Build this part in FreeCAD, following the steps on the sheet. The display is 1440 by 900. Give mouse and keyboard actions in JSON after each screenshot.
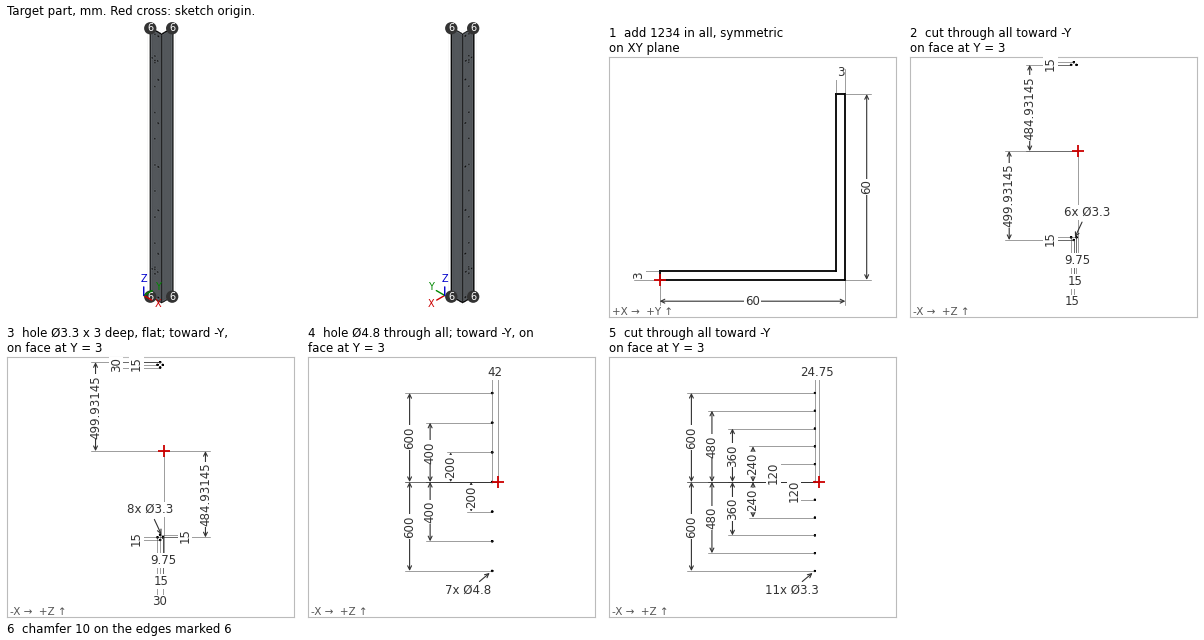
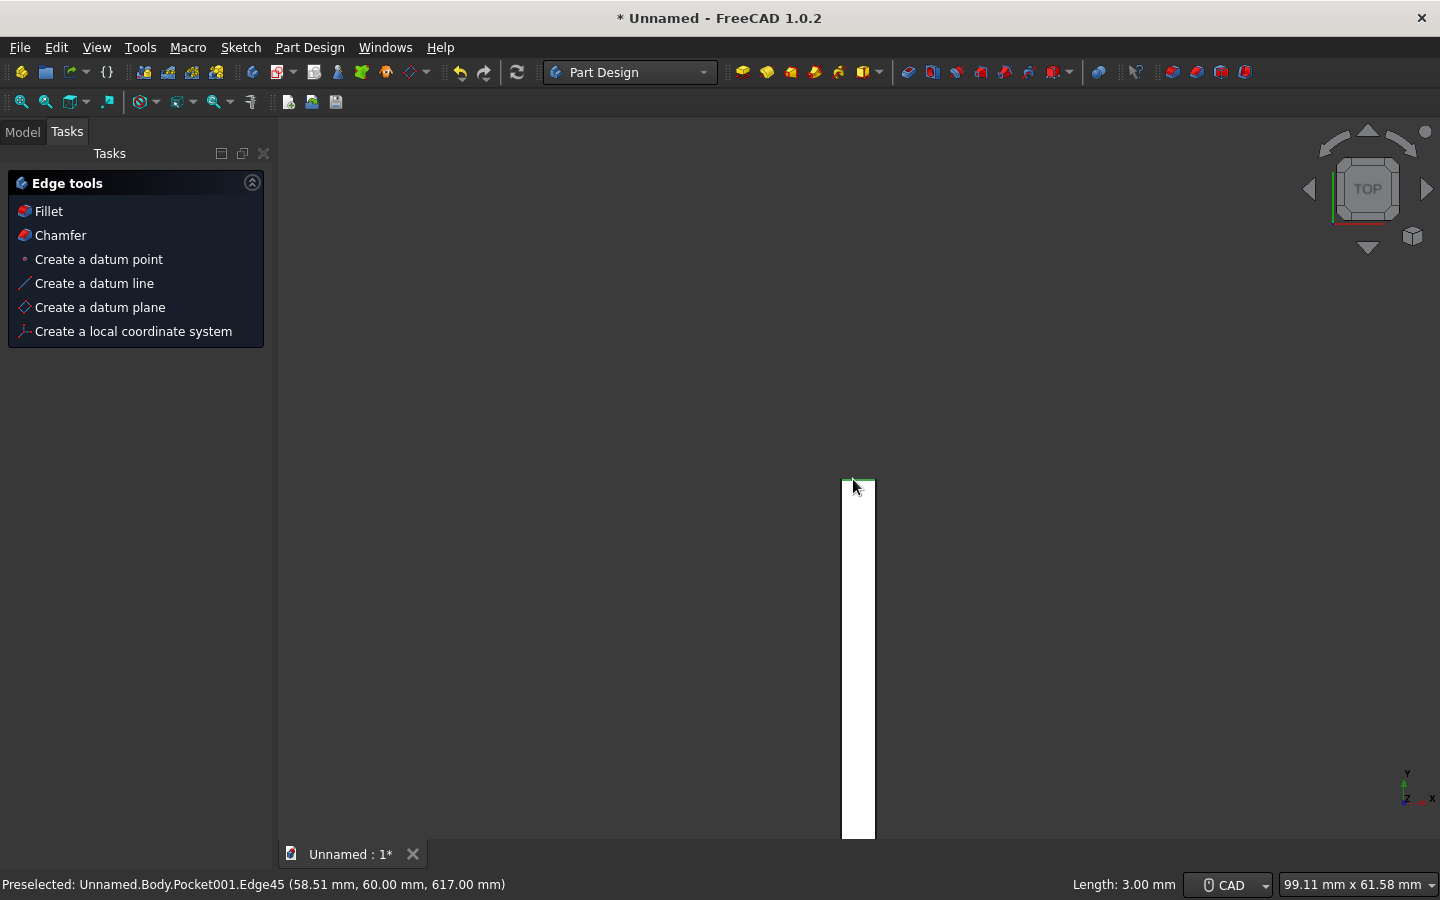
{"action": "left_click", "coordinate": [22, 102]}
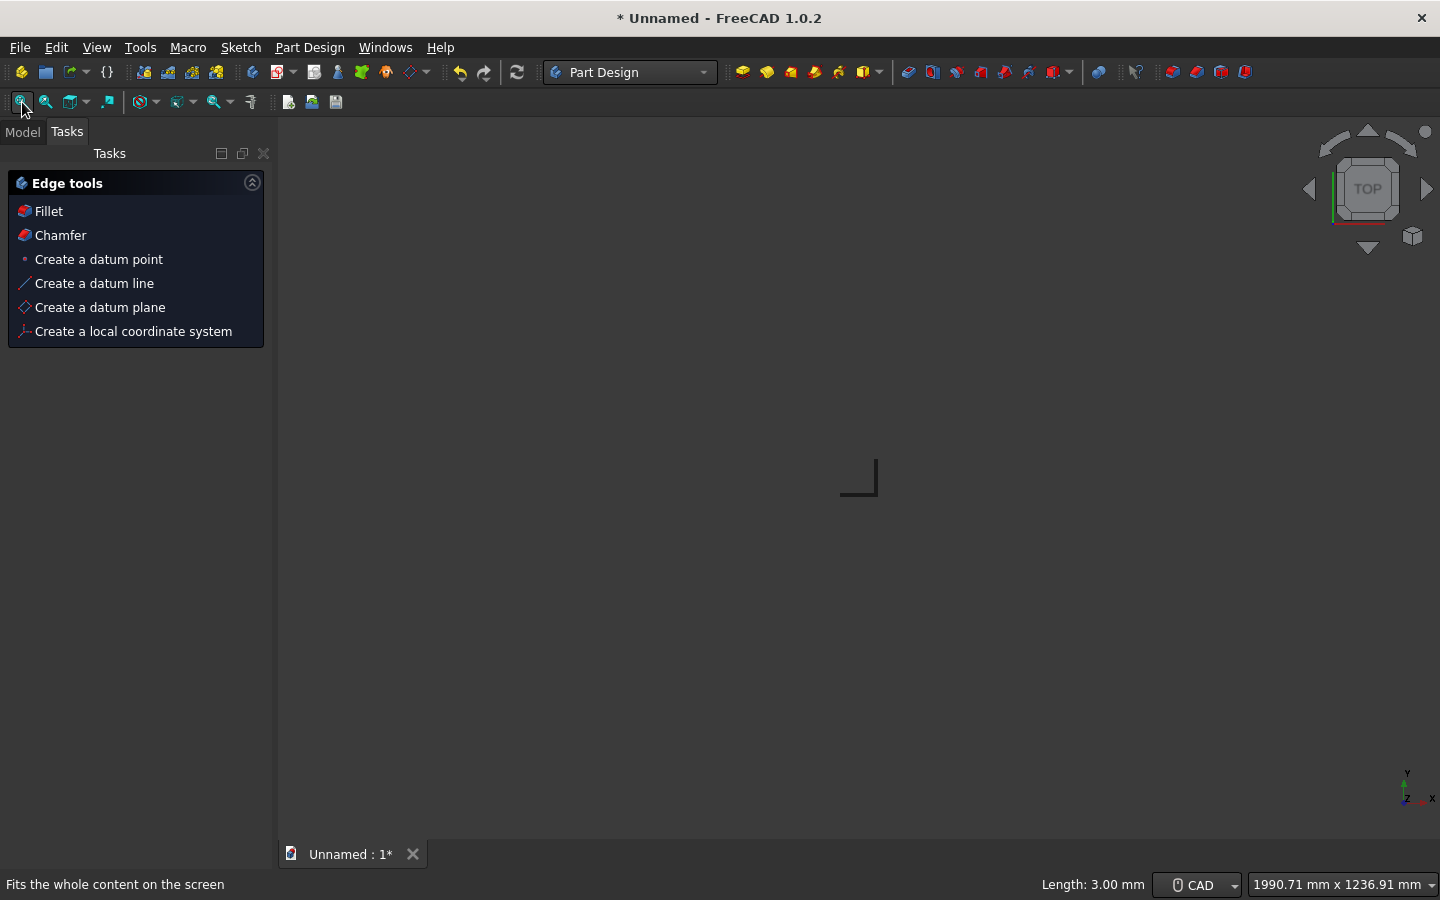
{"action": "key", "text": "1"}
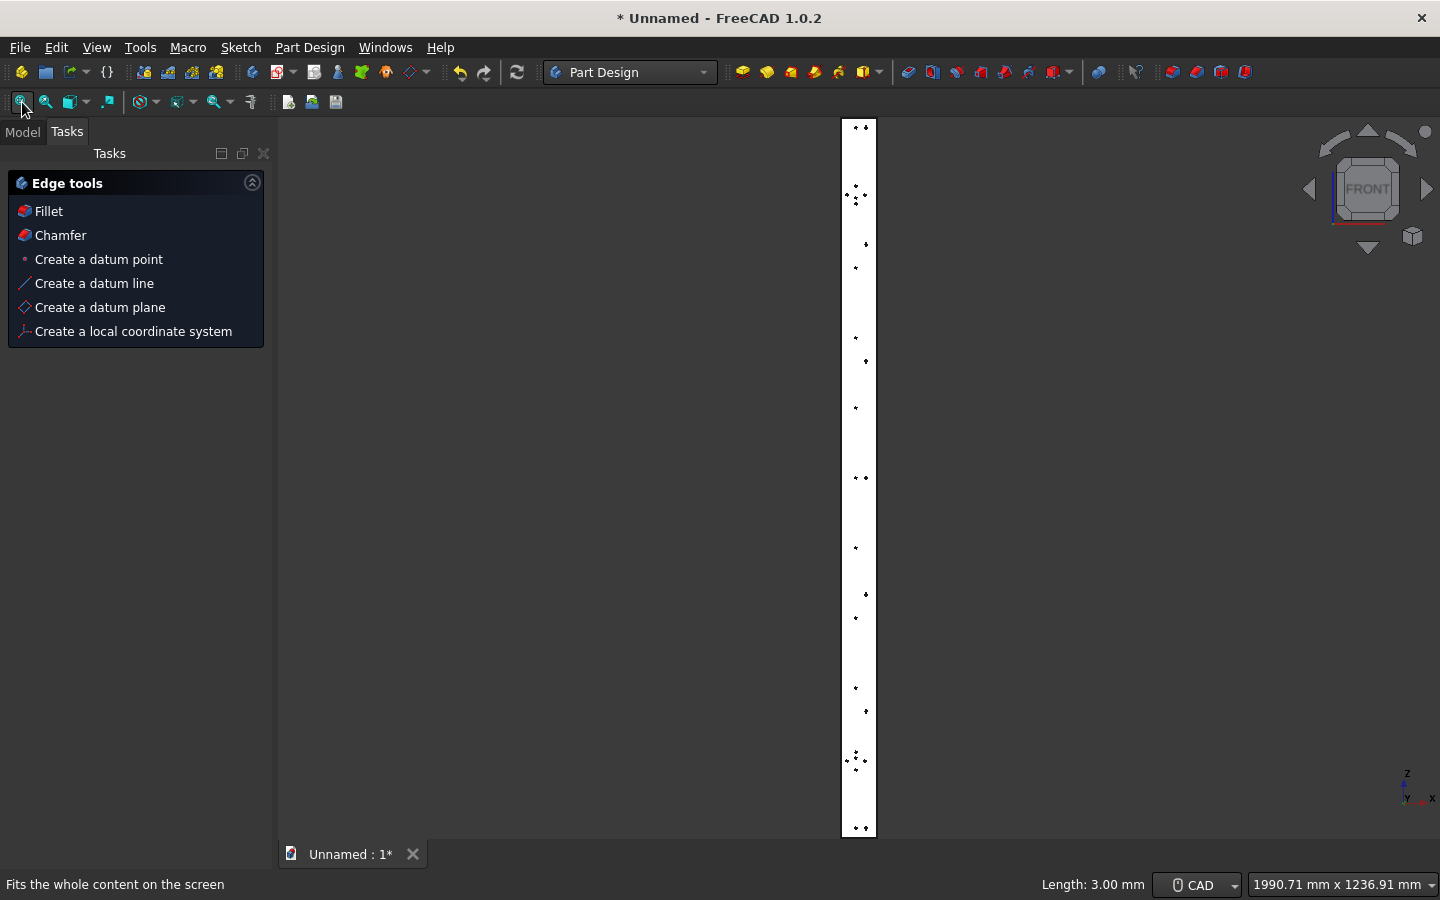
{"action": "key", "text": "3"}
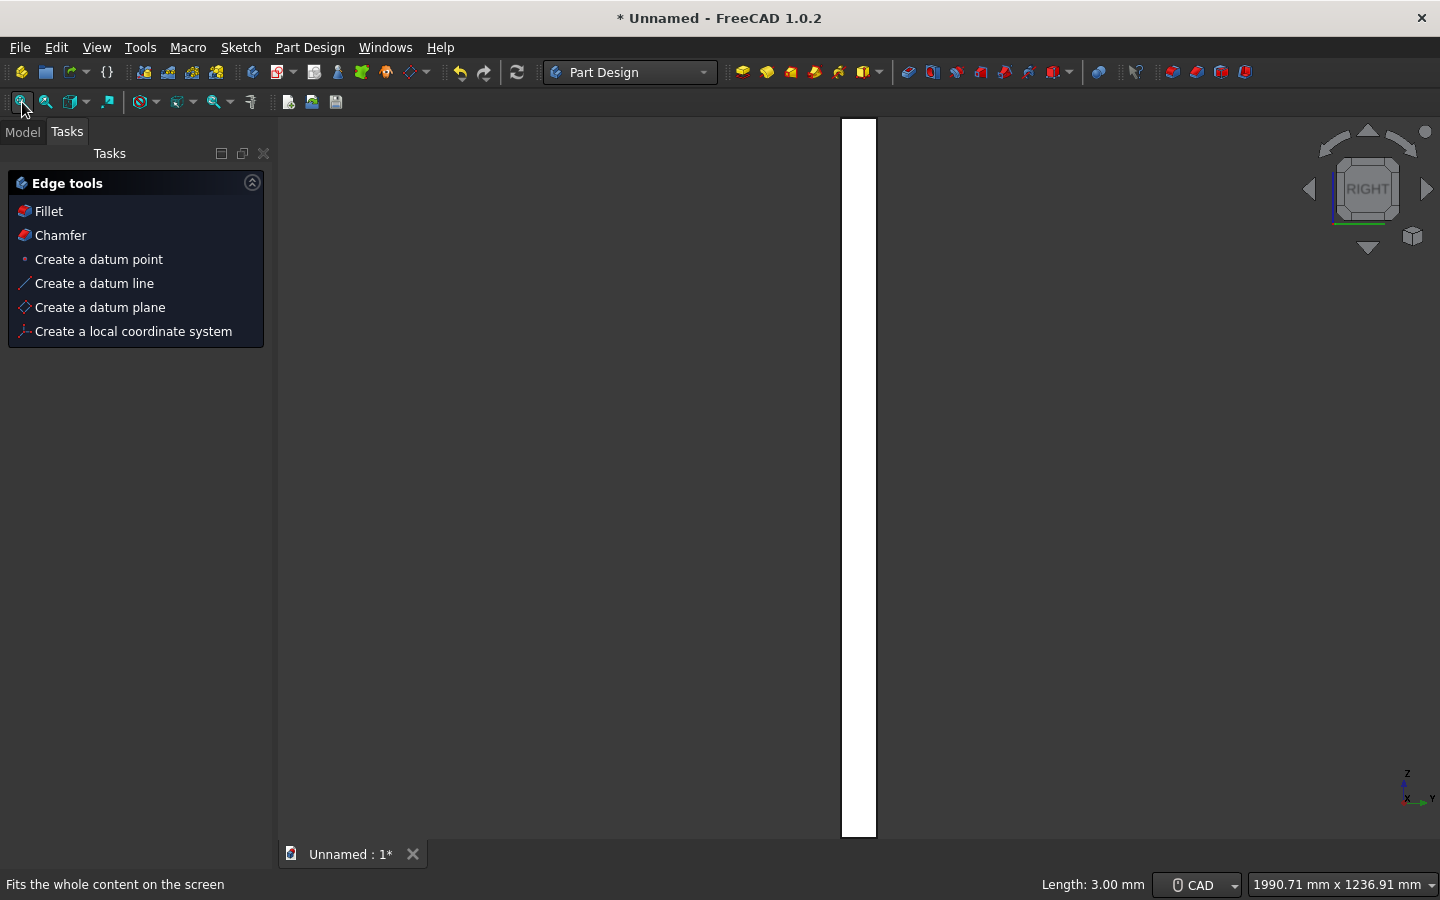
{"action": "key", "text": "5"}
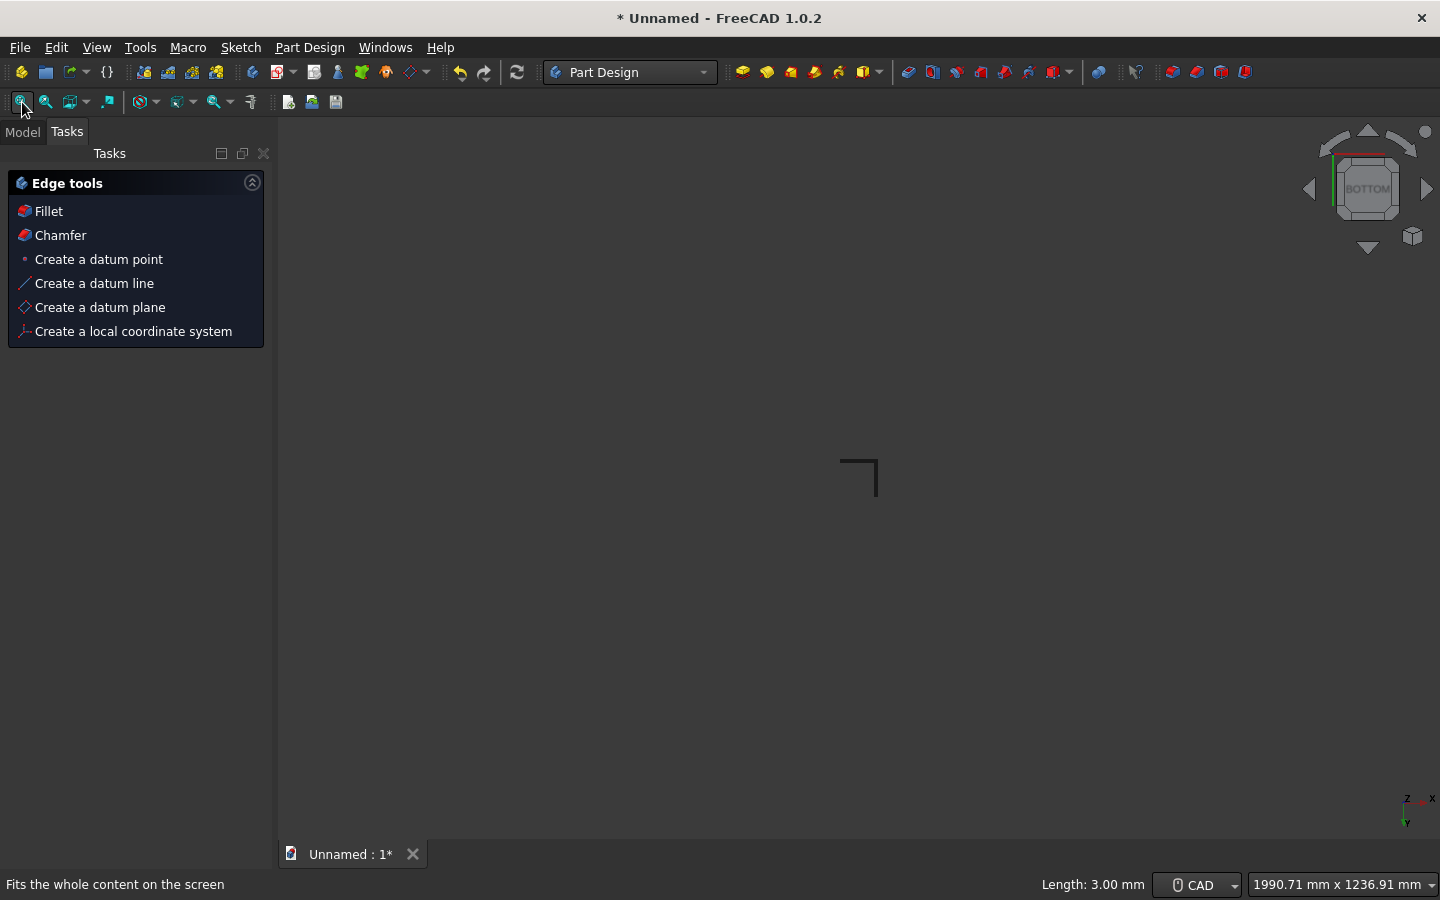
{"action": "left_click", "coordinate": [22, 102]}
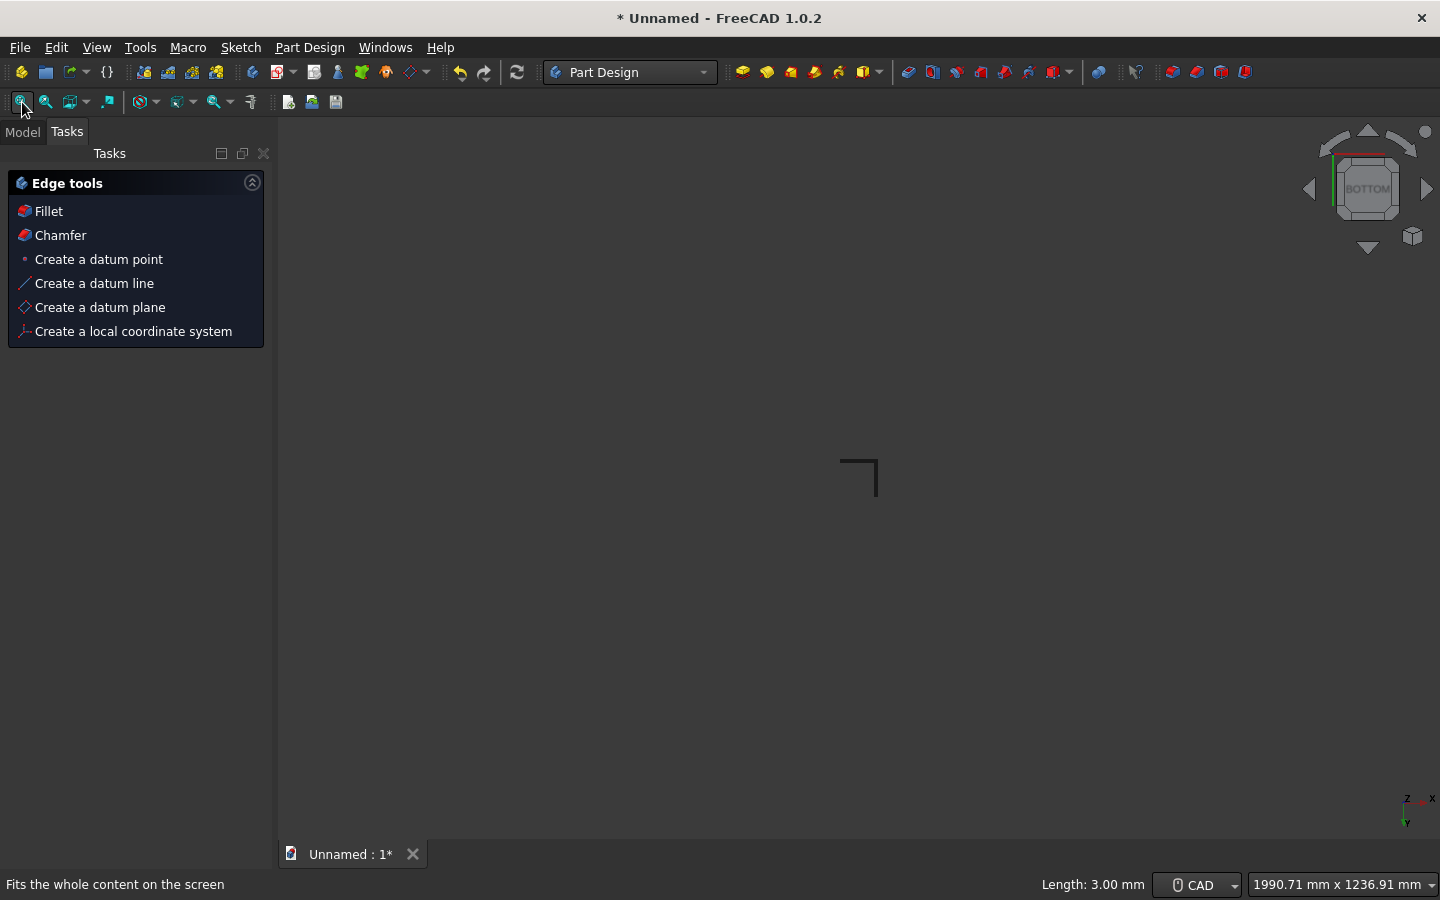
{"action": "scroll", "coordinate": [841, 460], "scroll_direction": "up", "scroll_amount": 15}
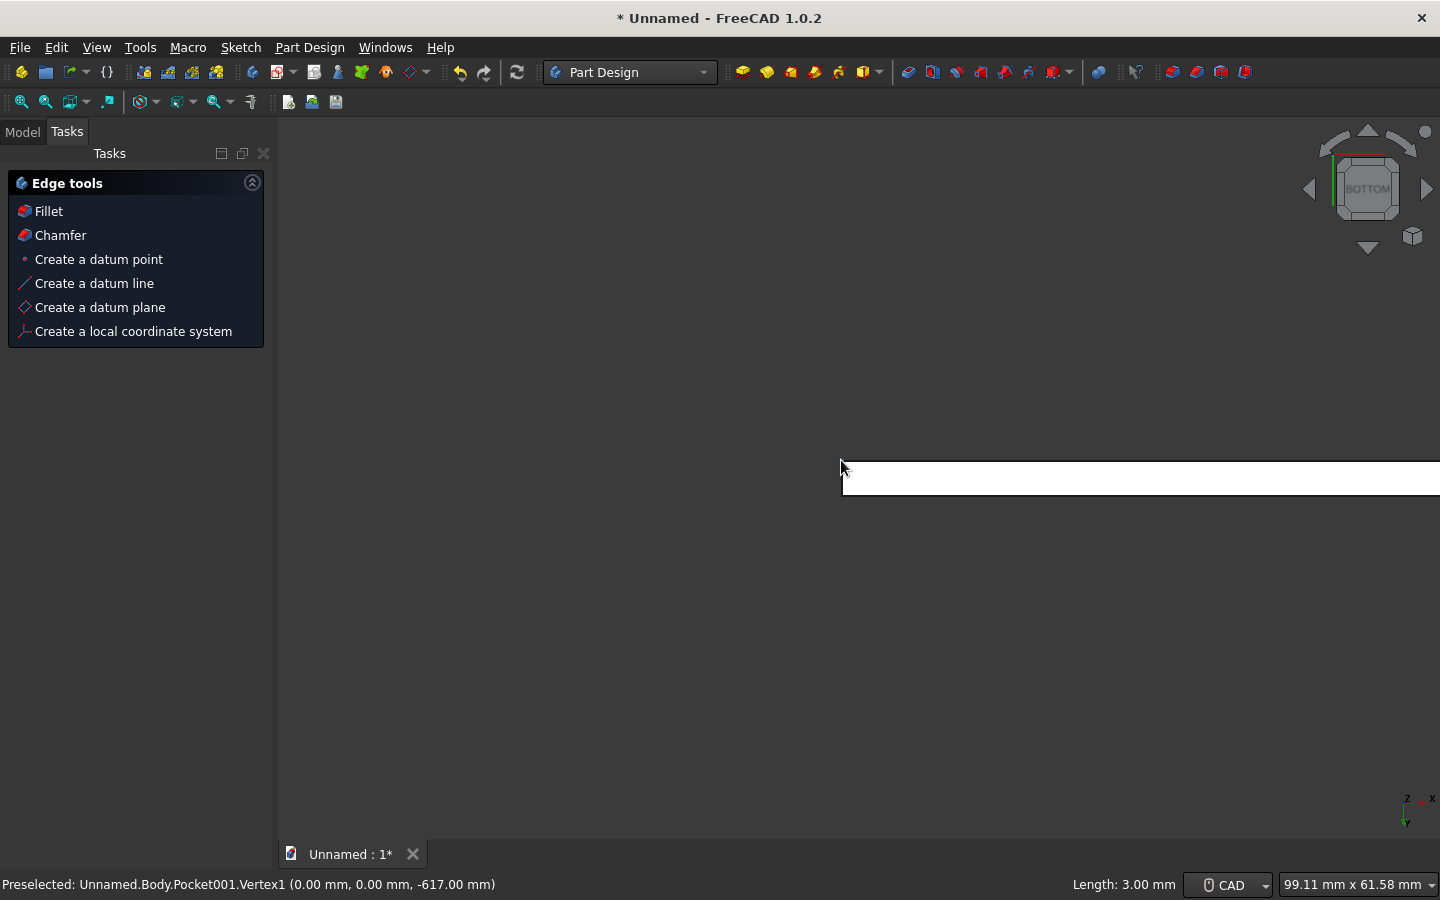
{"action": "left_click", "coordinate": [842, 477], "text": "ctrl"}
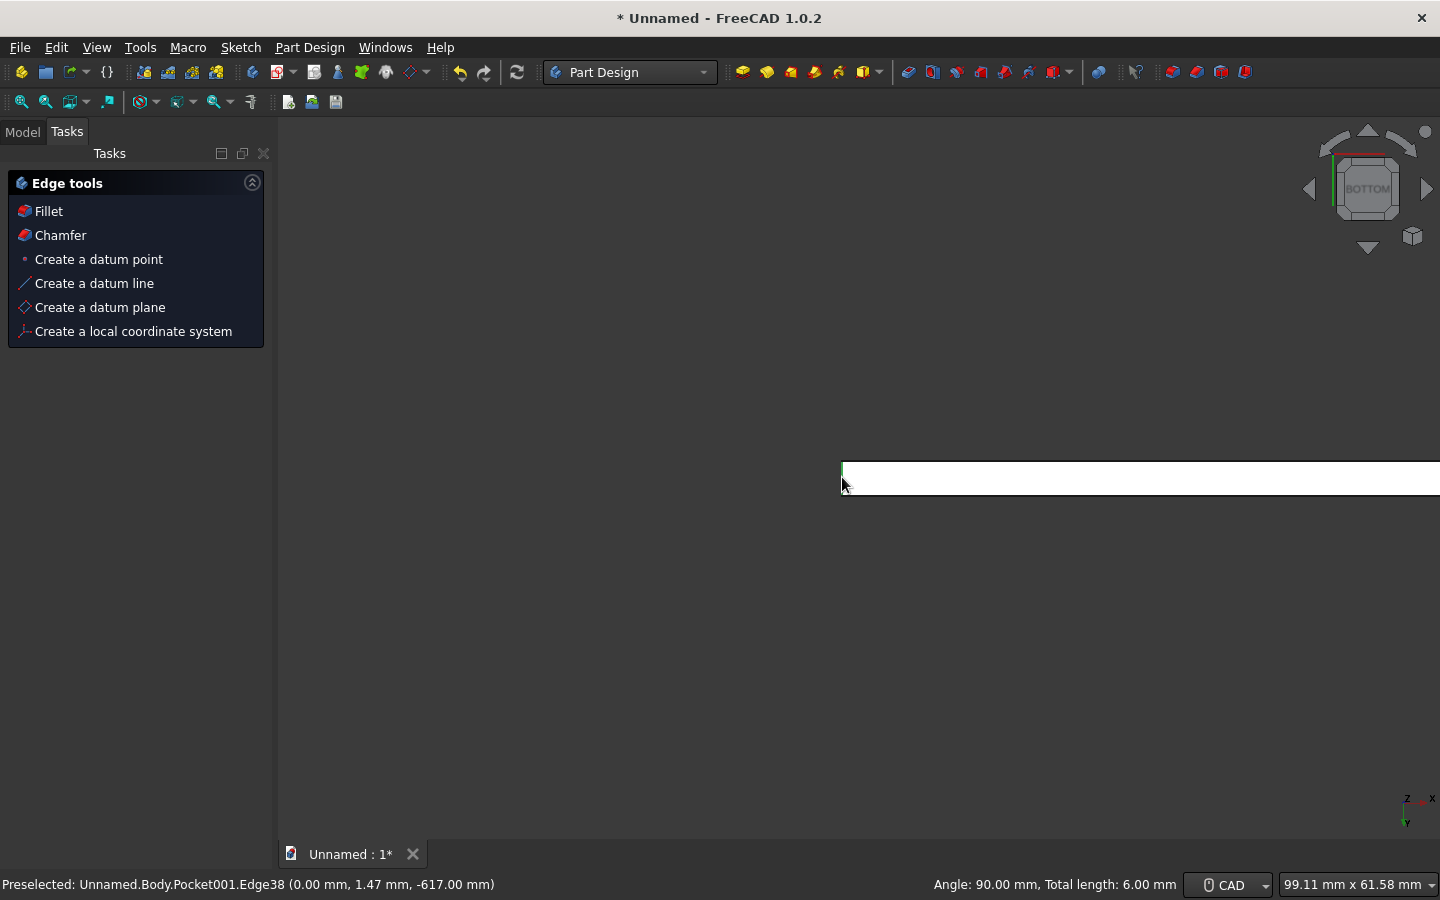
{"action": "left_click", "coordinate": [22, 102]}